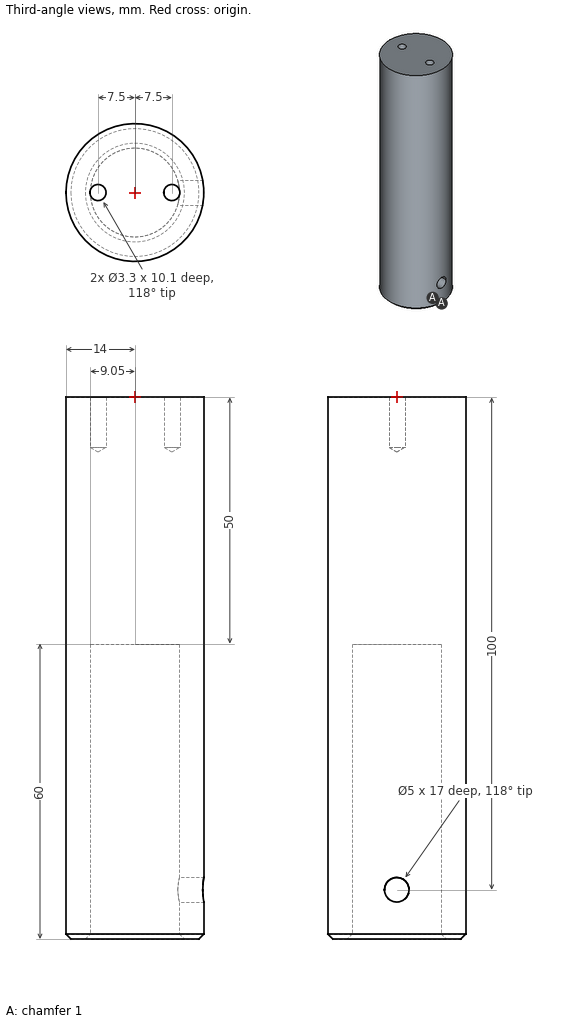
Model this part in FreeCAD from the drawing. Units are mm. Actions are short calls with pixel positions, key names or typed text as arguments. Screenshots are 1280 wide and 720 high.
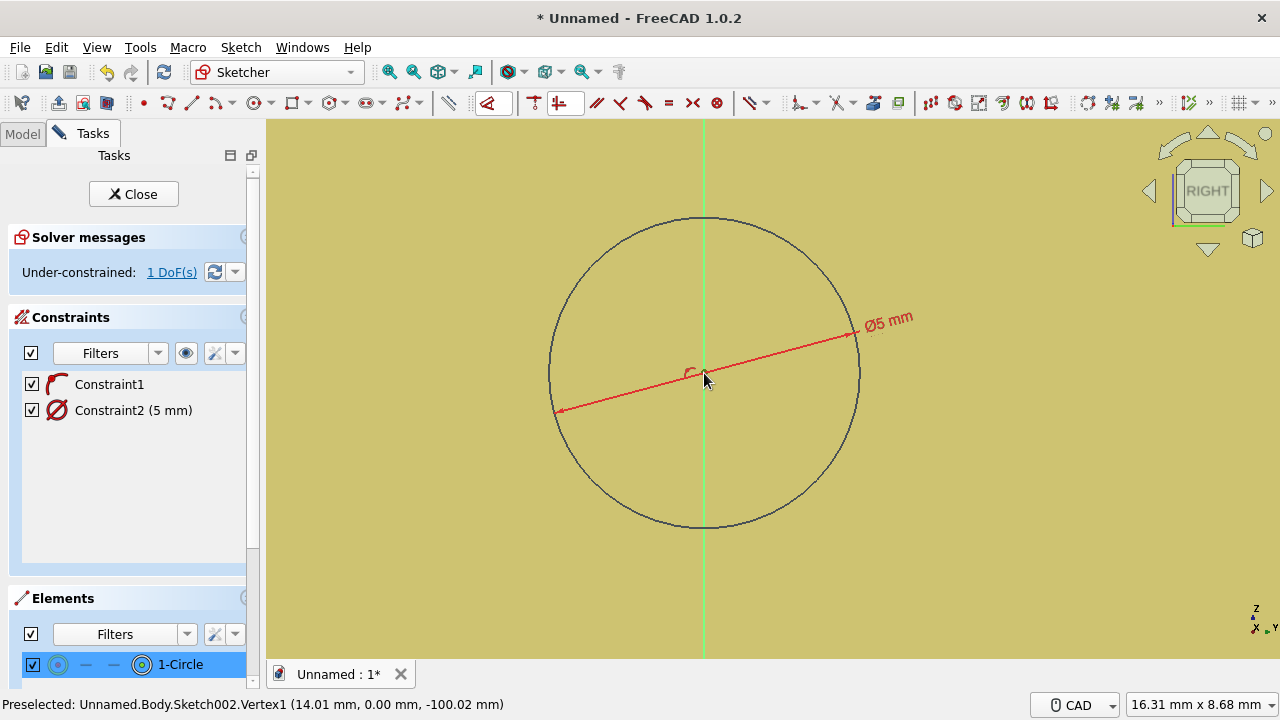
click(506, 104)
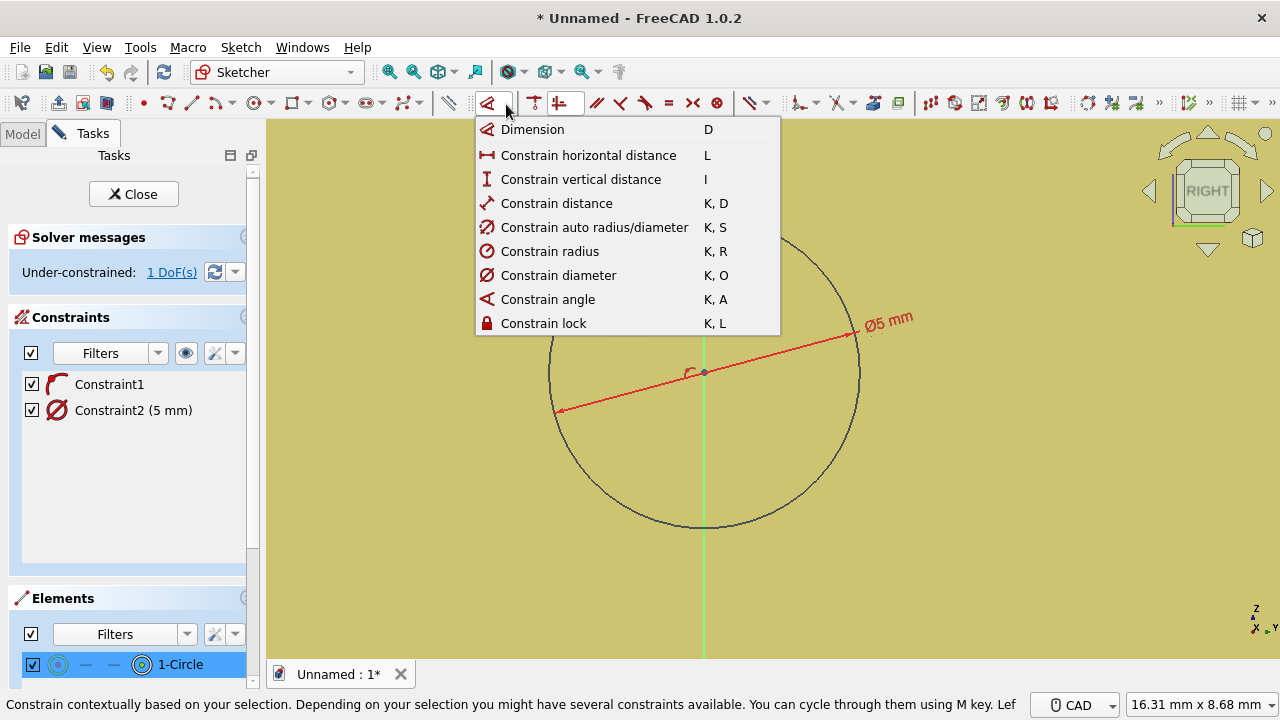
click(628, 179)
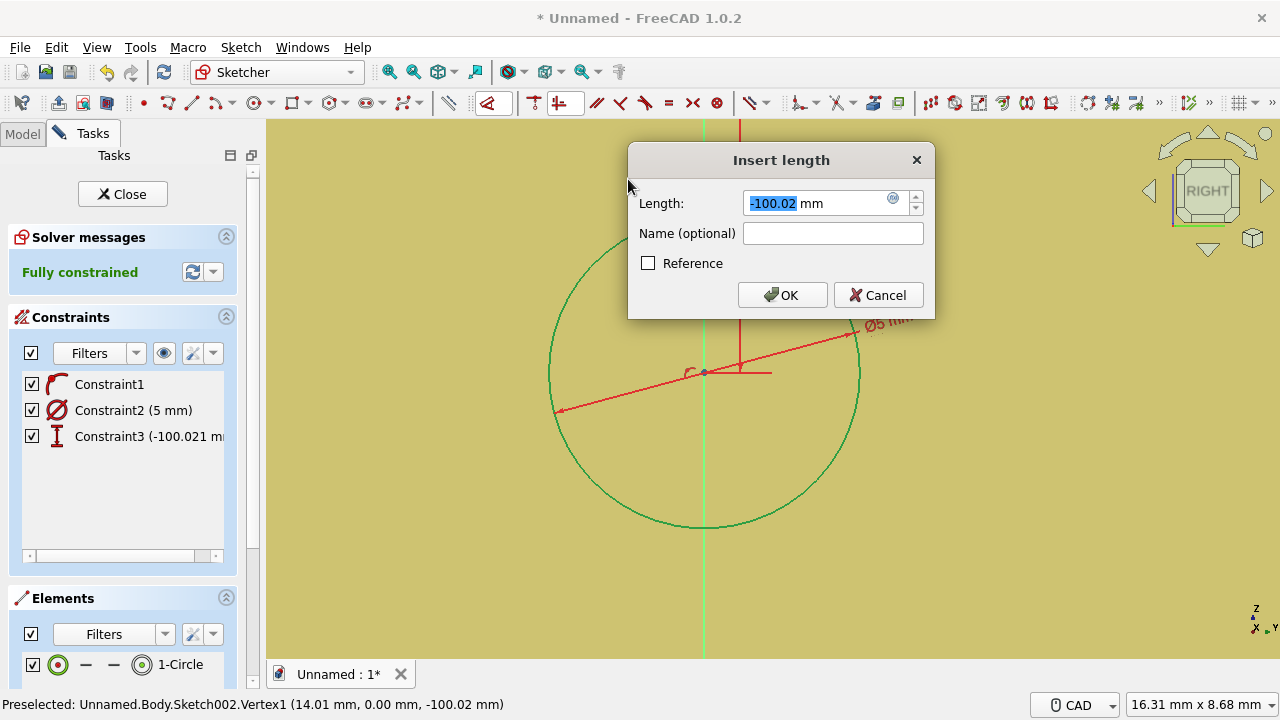
text(-100)
key(Return)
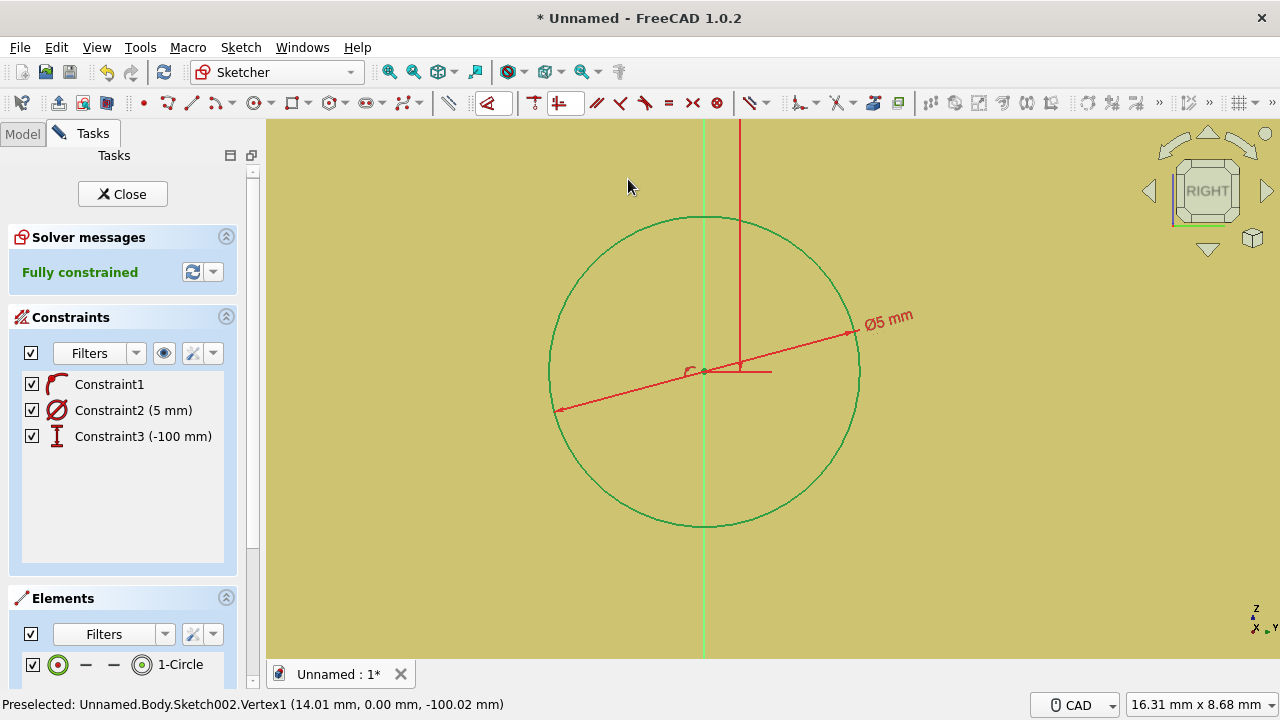
click(123, 194)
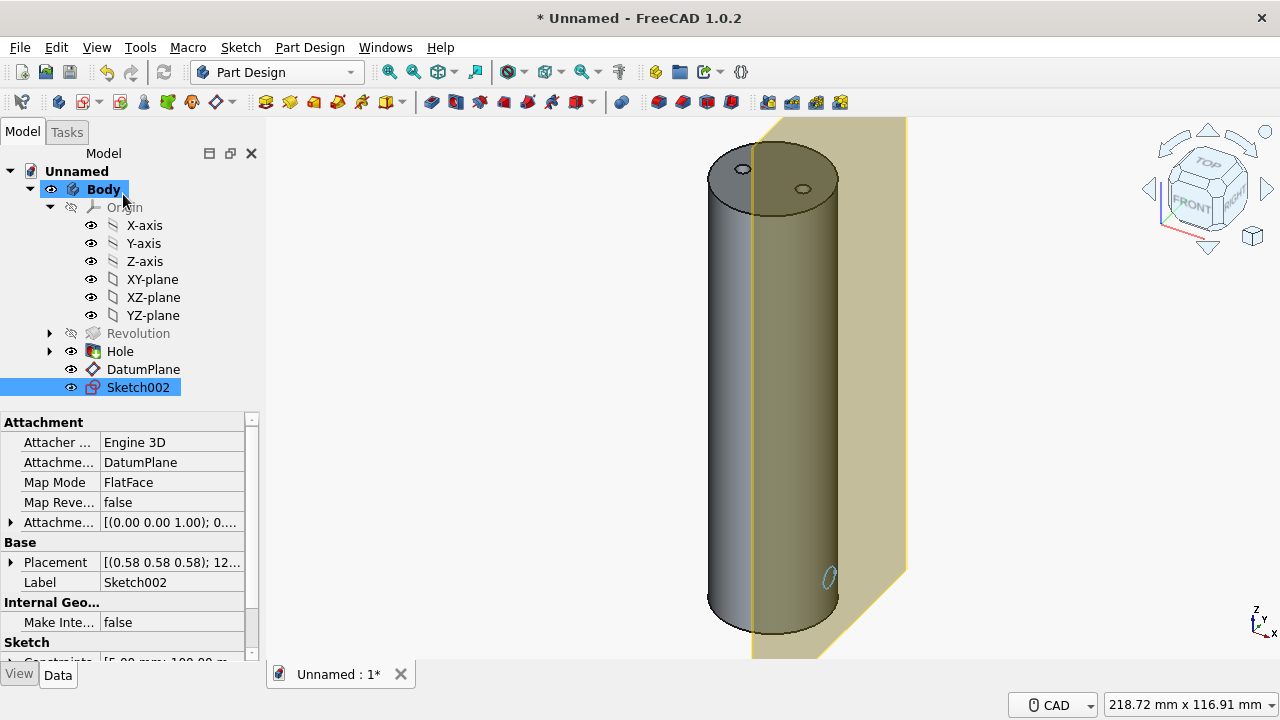
click(456, 102)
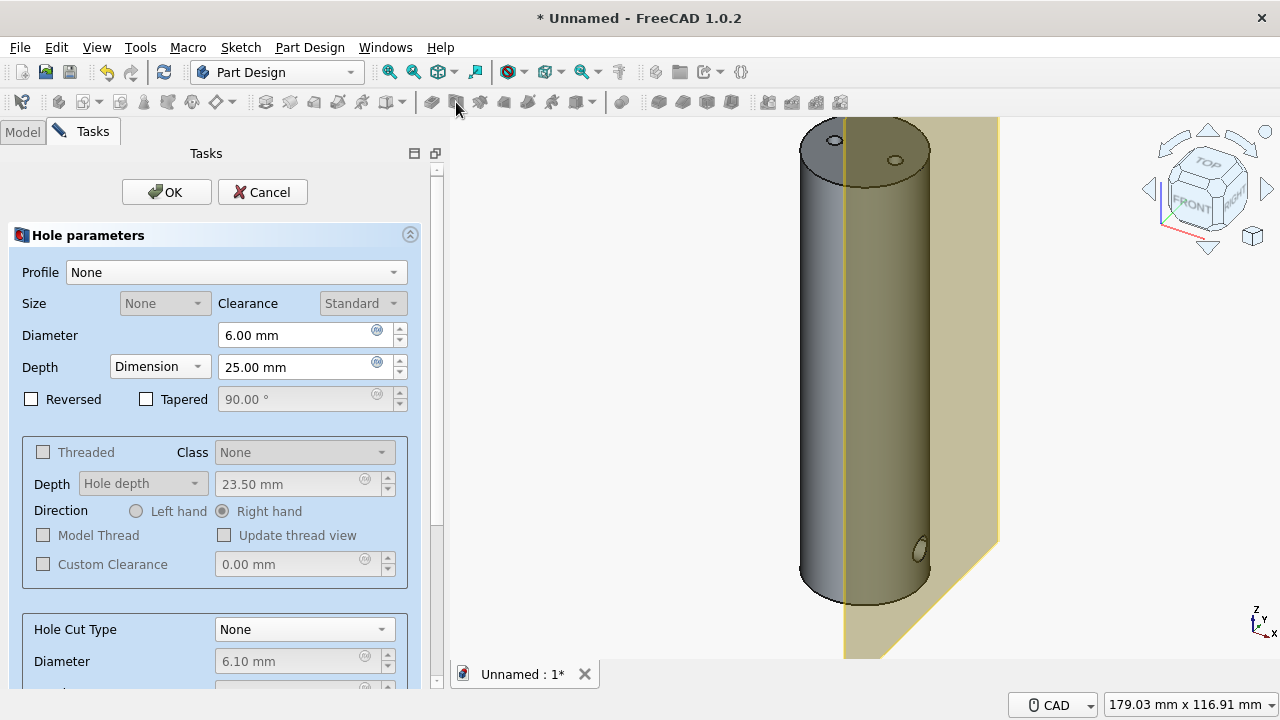
triple_click(305, 335)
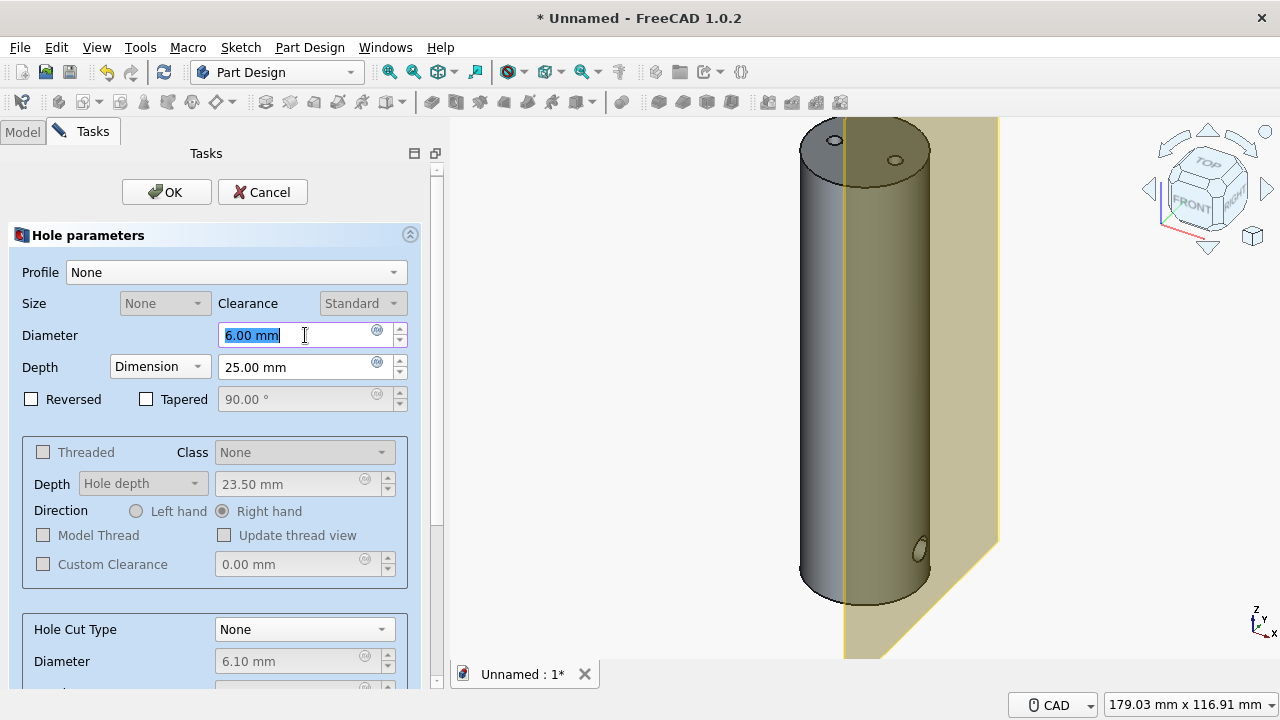
text(5)
key(Tab)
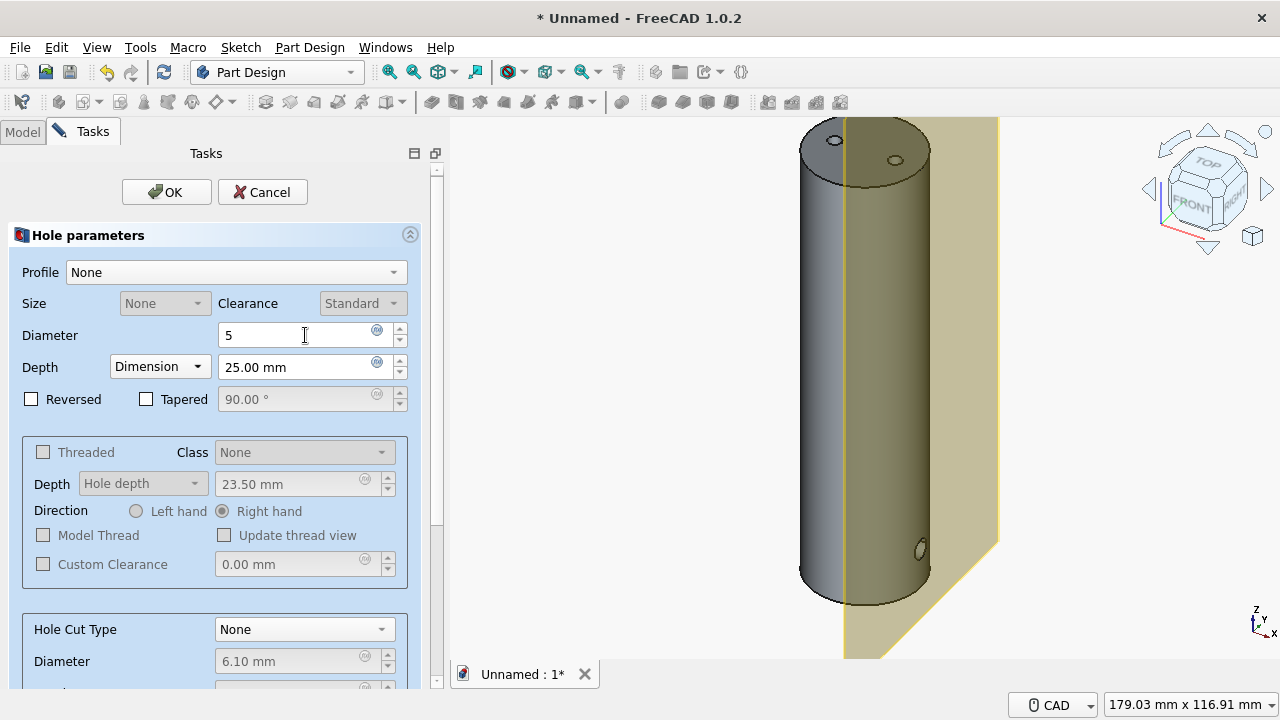
triple_click(305, 367)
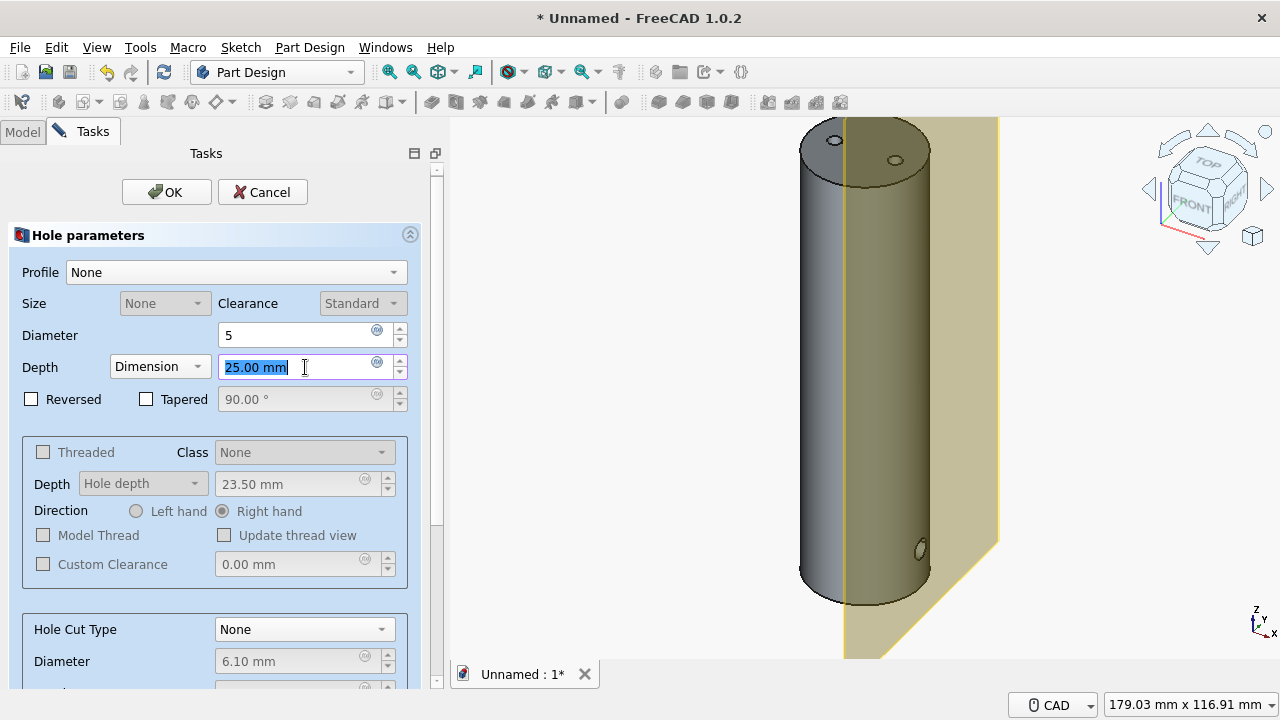
text(17)
key(Tab)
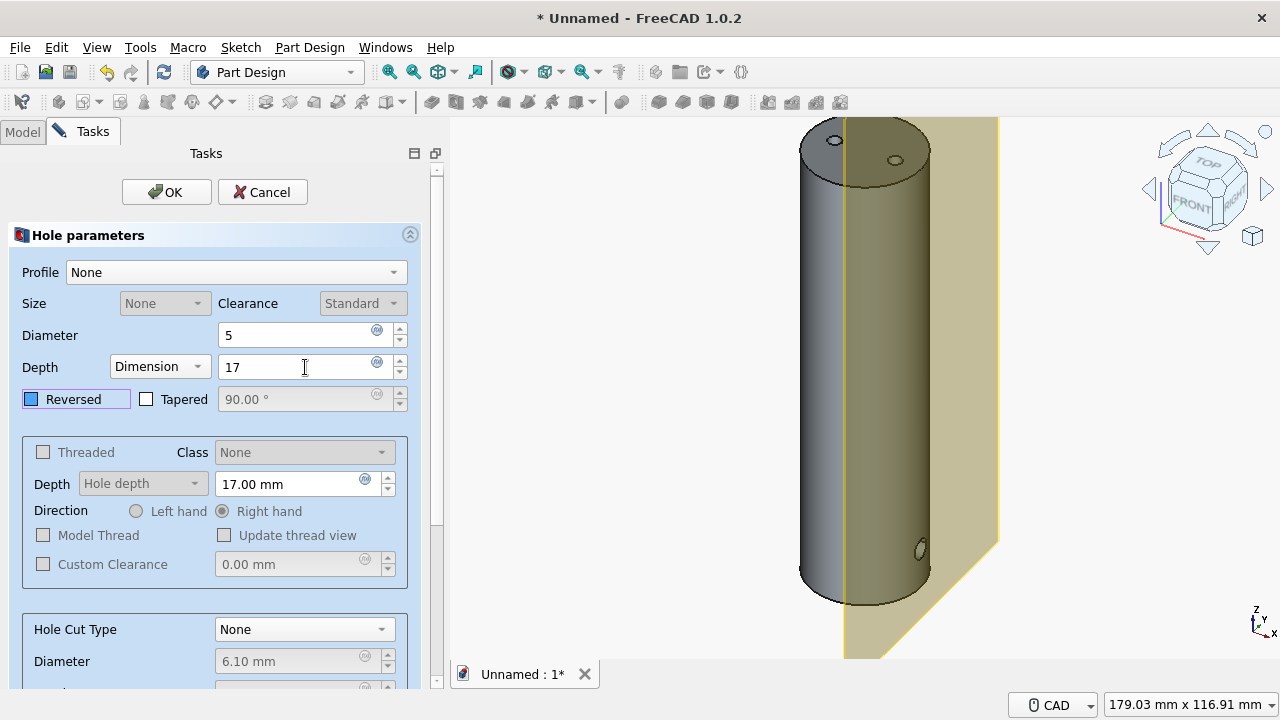
click(167, 192)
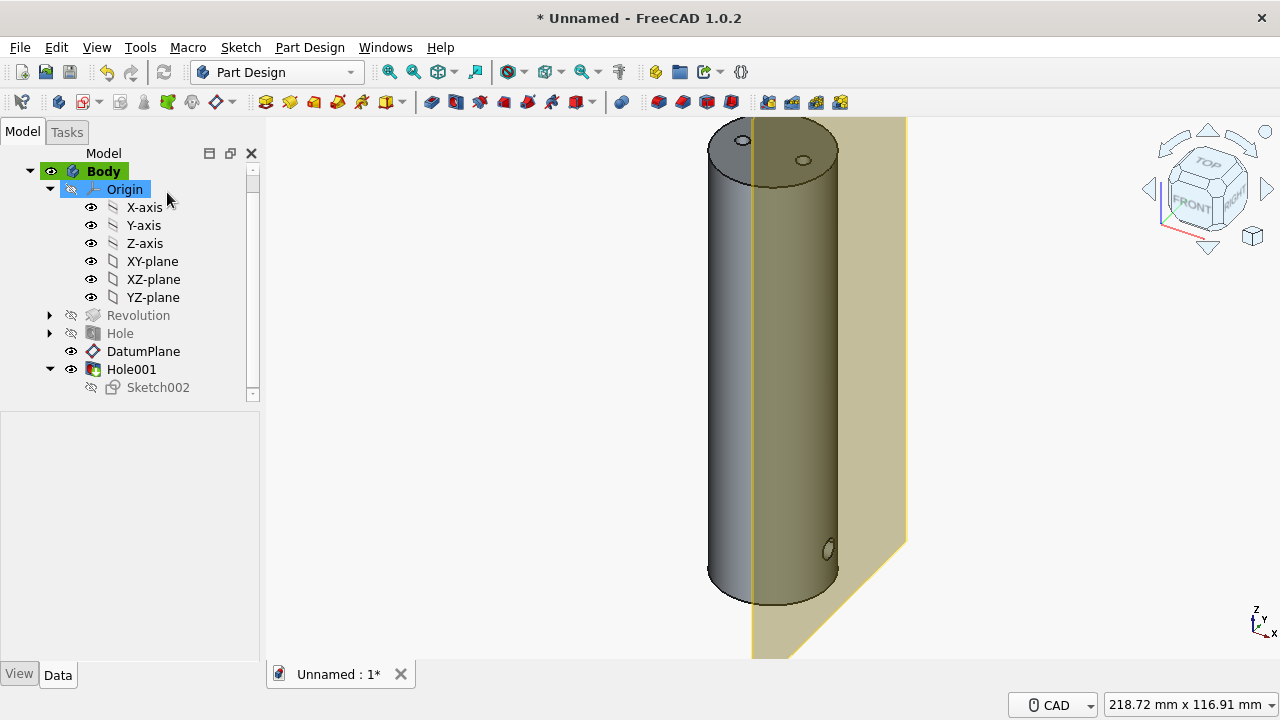
click(116, 351)
key(space)